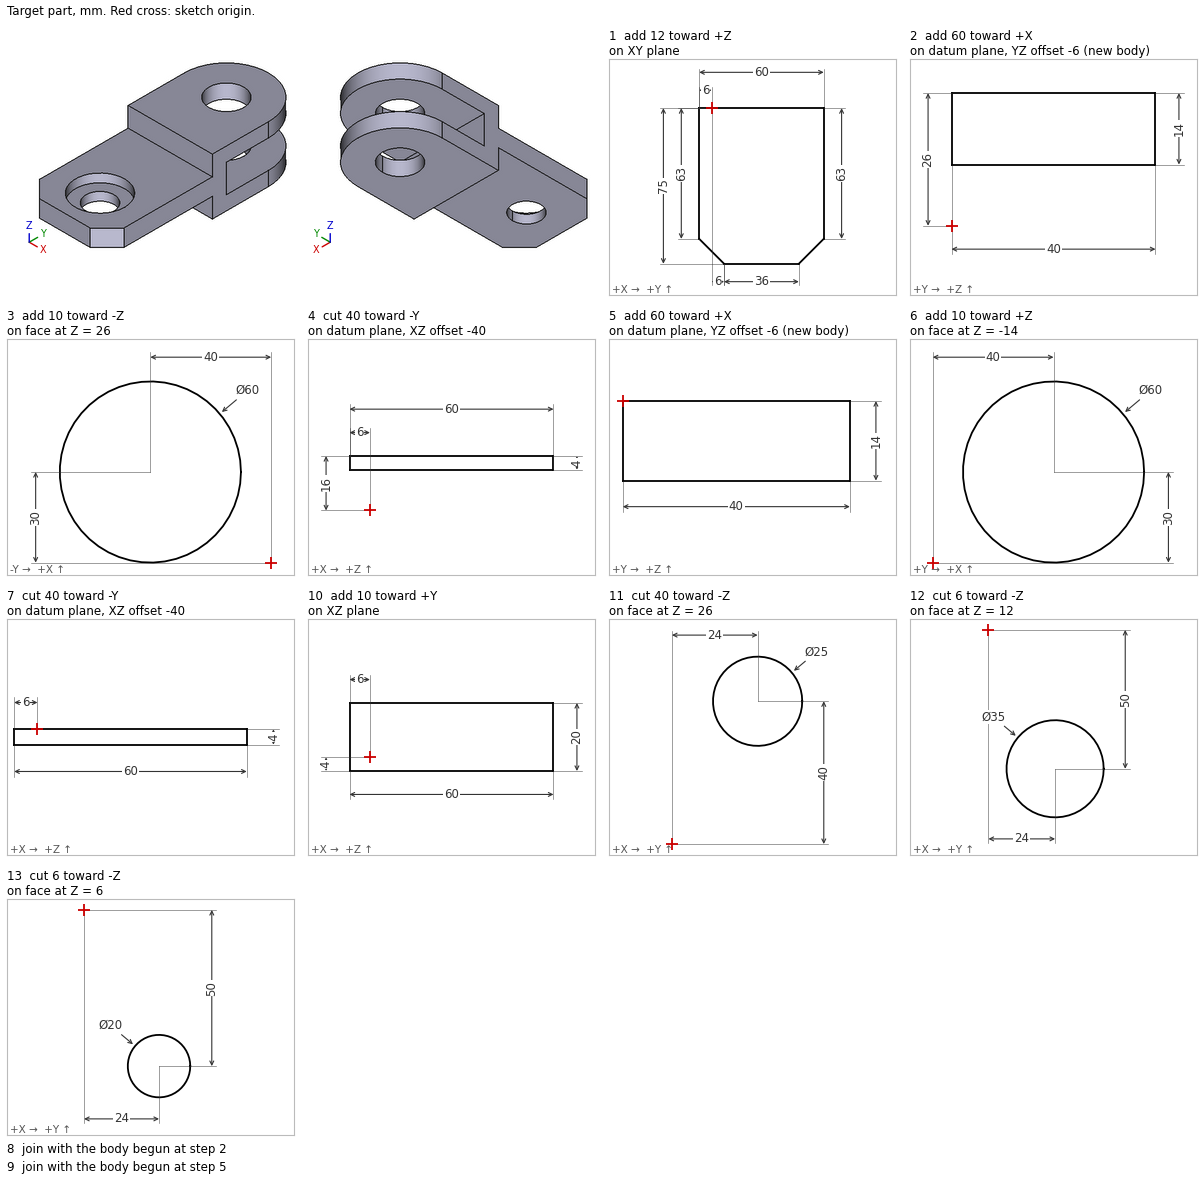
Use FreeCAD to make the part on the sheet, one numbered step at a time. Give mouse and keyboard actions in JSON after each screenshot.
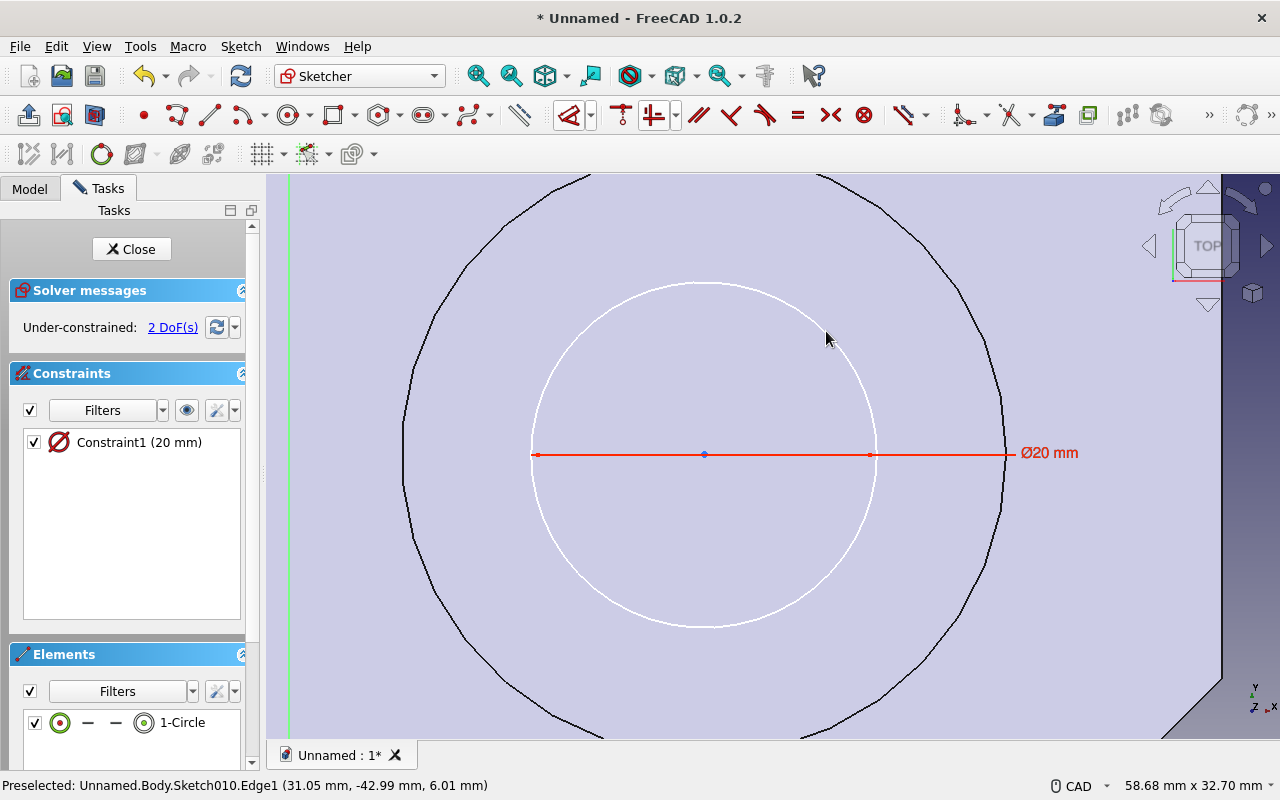
{"action": "left_click", "coordinate": [704, 455]}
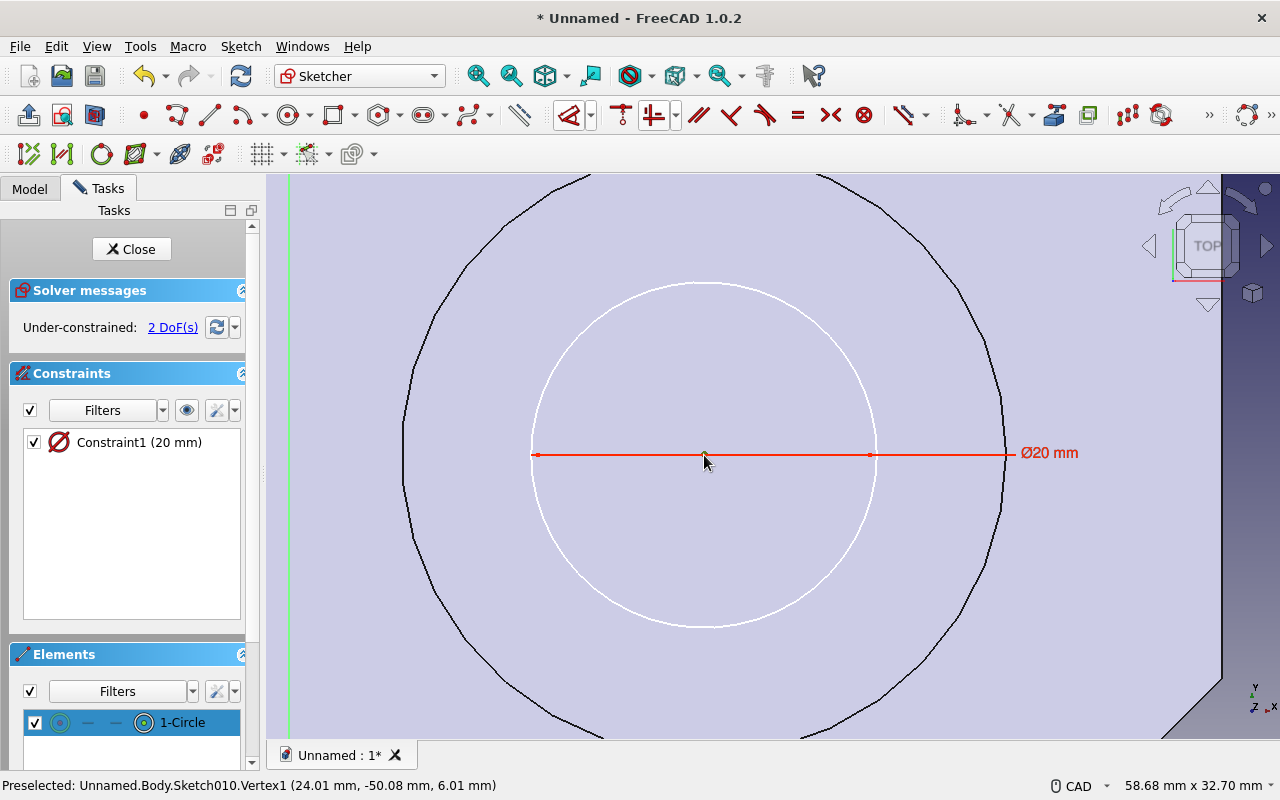
{"action": "left_click", "coordinate": [590, 116]}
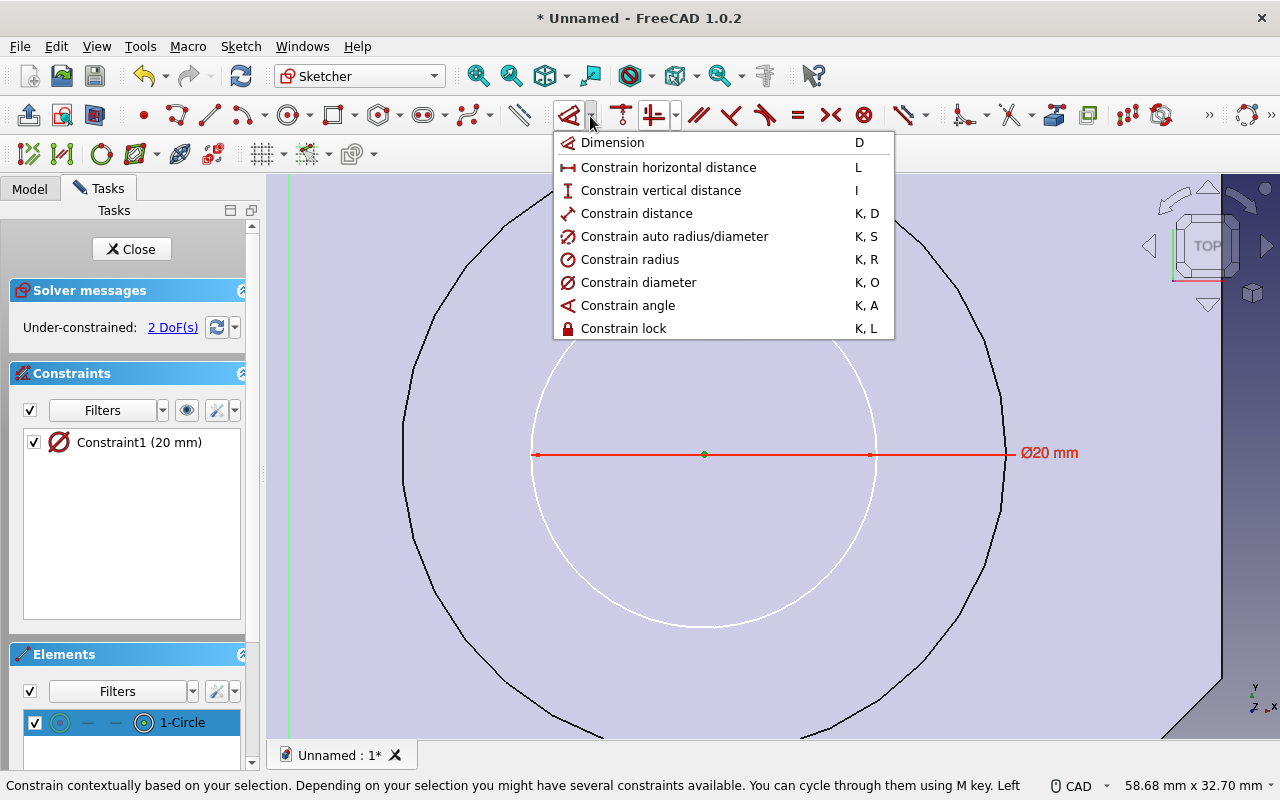
{"action": "left_click", "coordinate": [724, 168]}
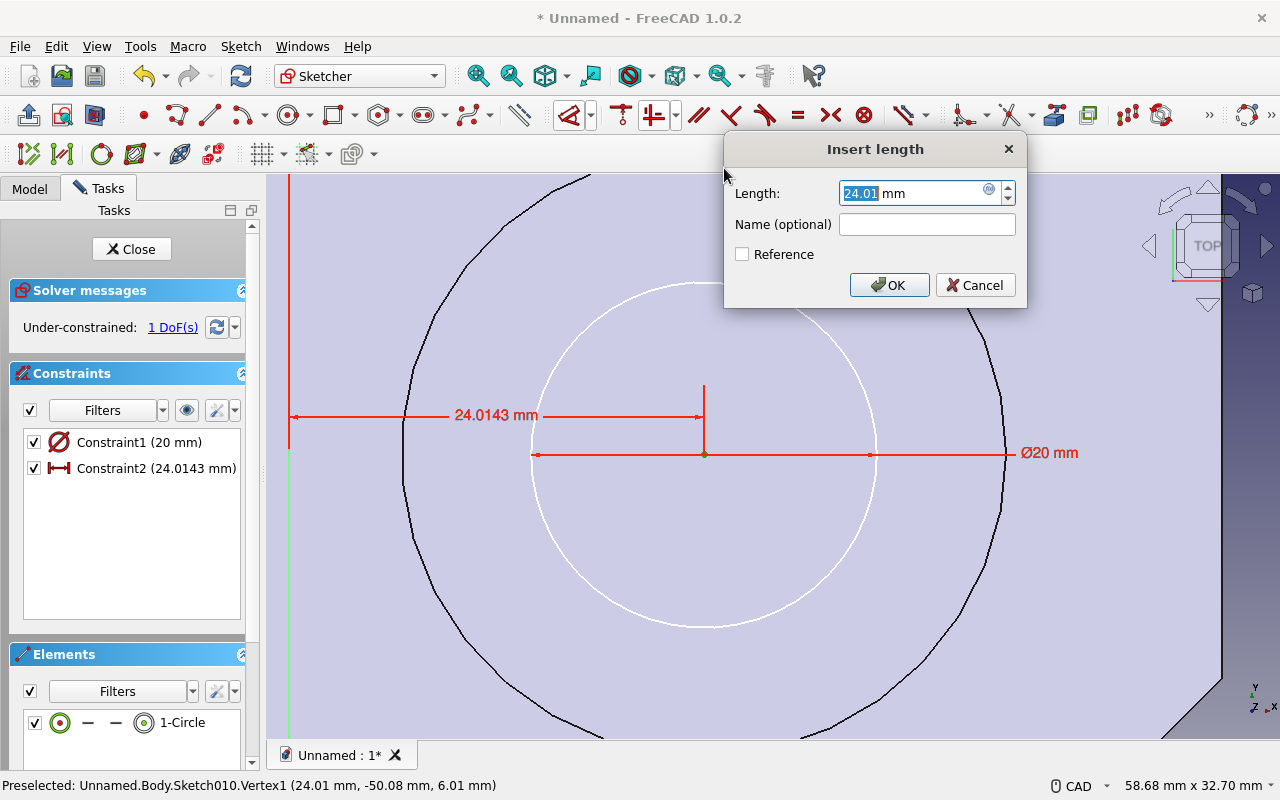
{"action": "type", "text": "24"}
{"action": "key", "text": "Return"}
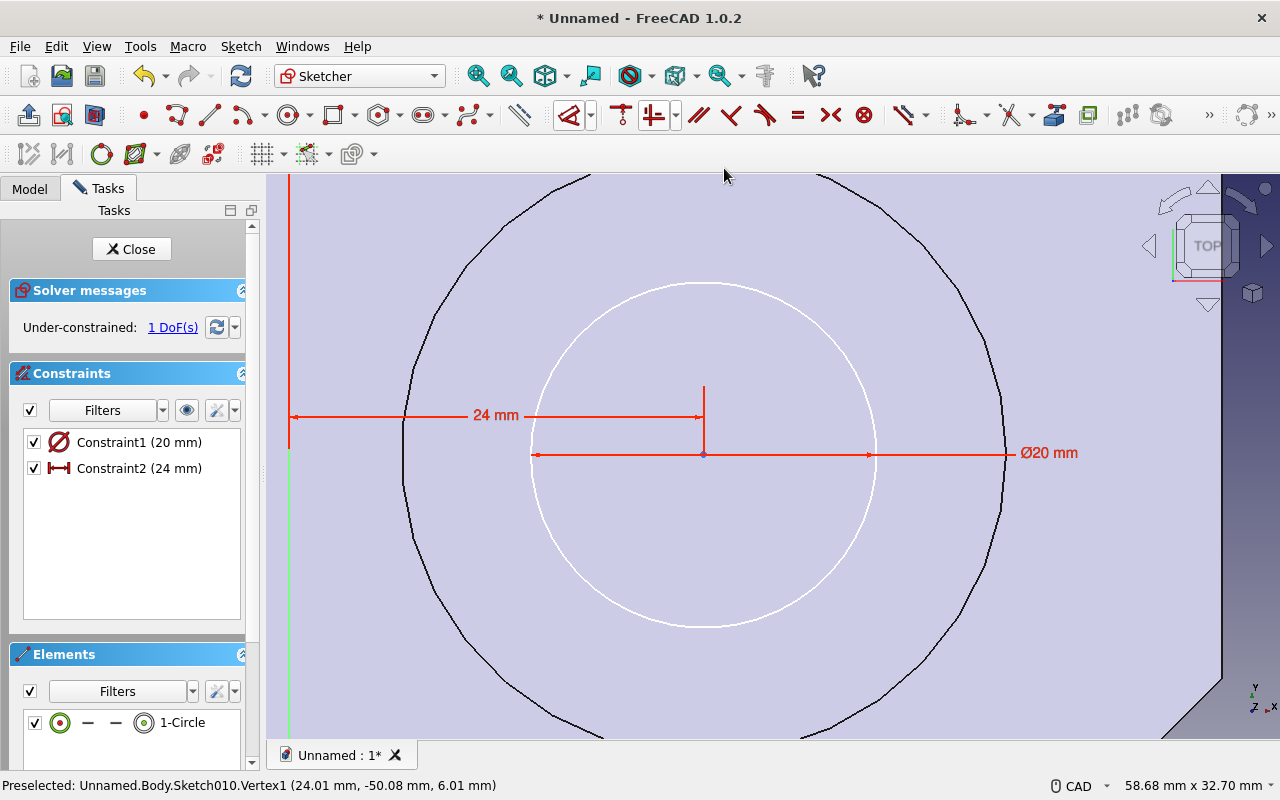
{"action": "left_click", "coordinate": [704, 455]}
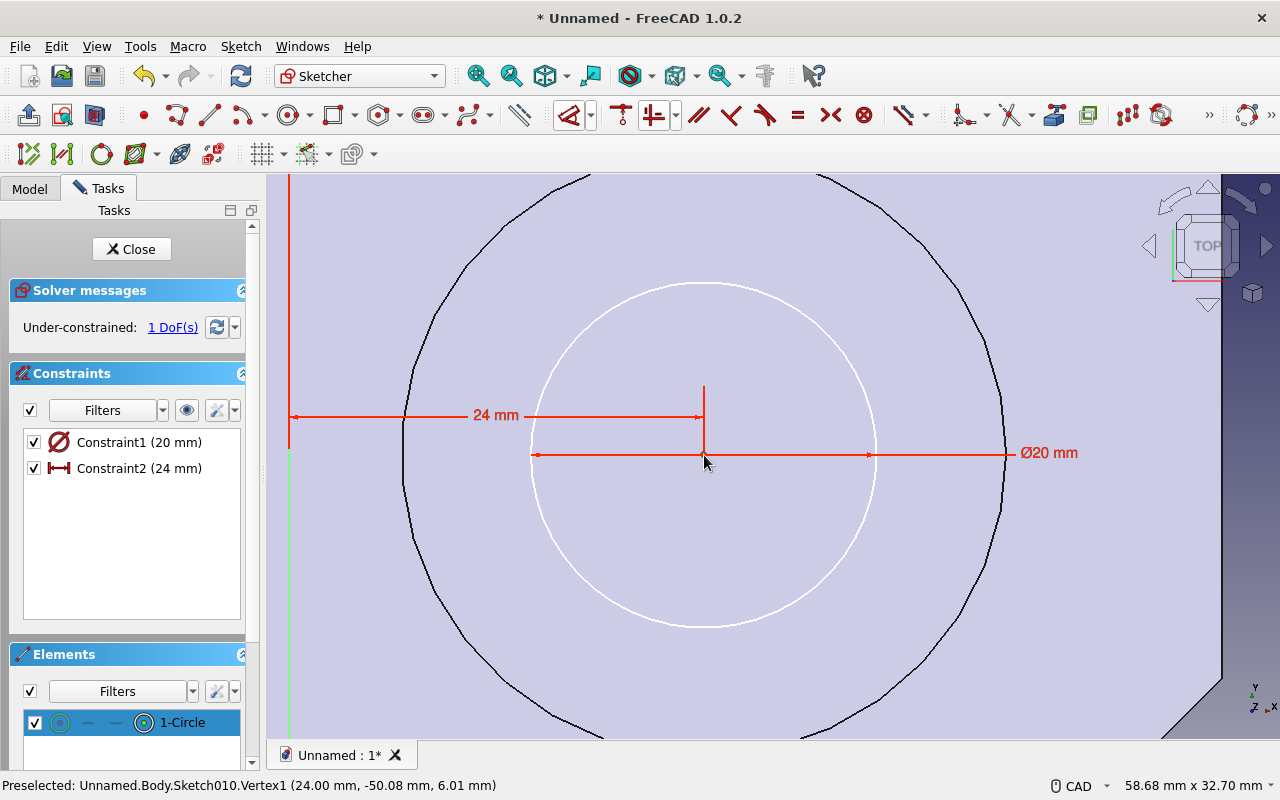
{"action": "left_click", "coordinate": [590, 116]}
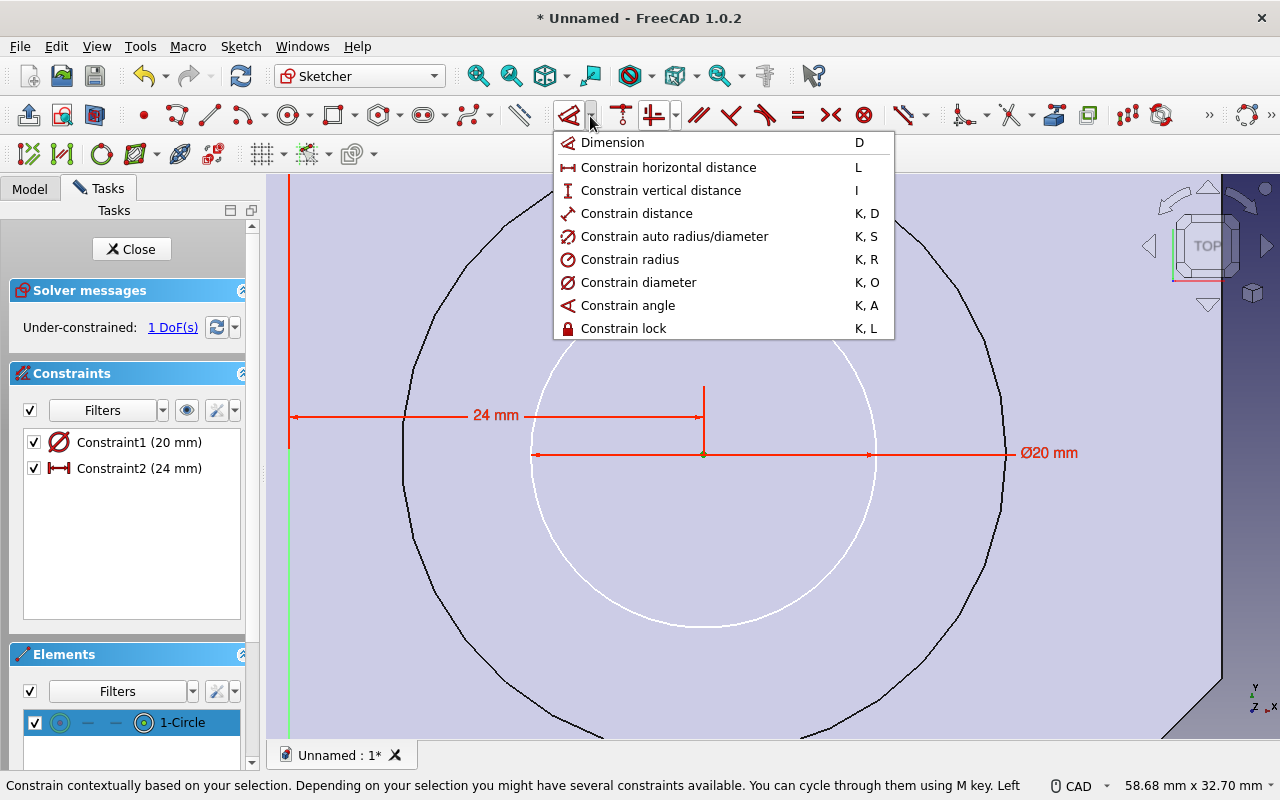
{"action": "left_click", "coordinate": [724, 190]}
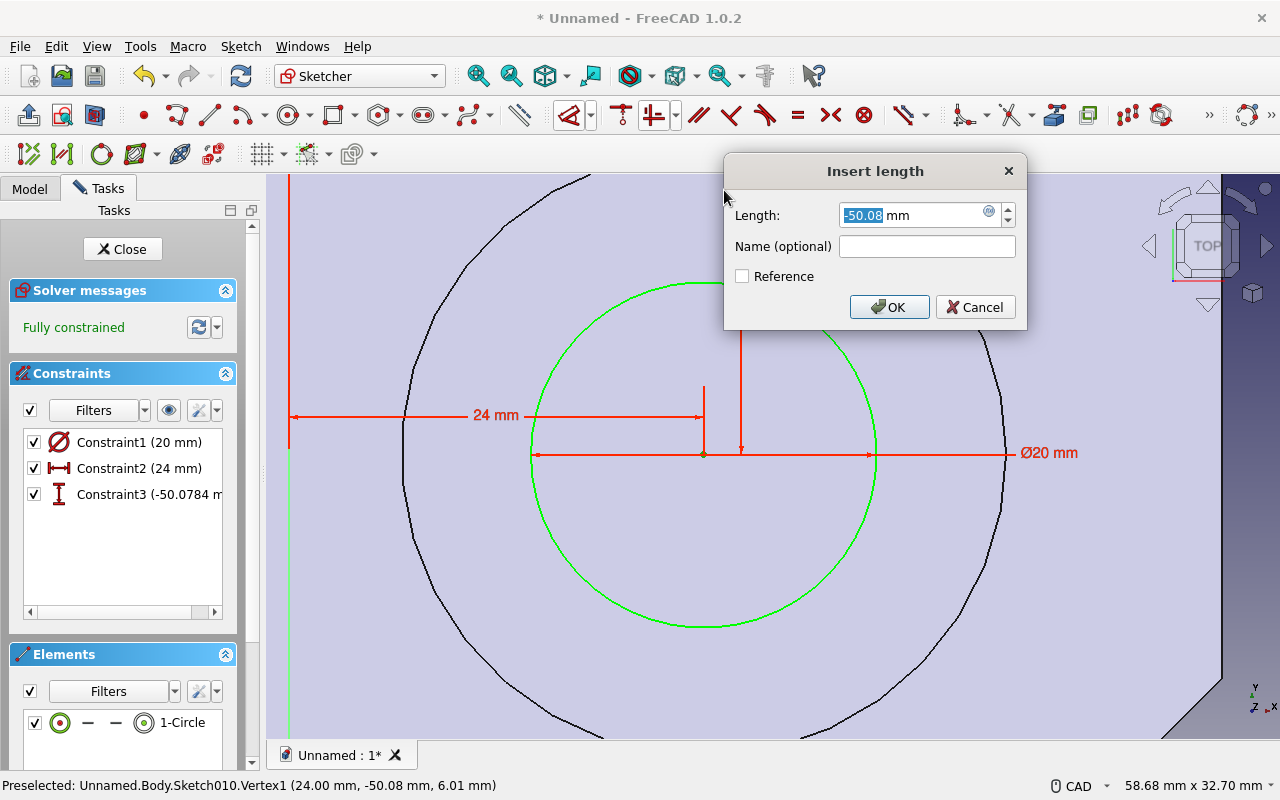
{"action": "type", "text": "-50"}
{"action": "key", "text": "Return"}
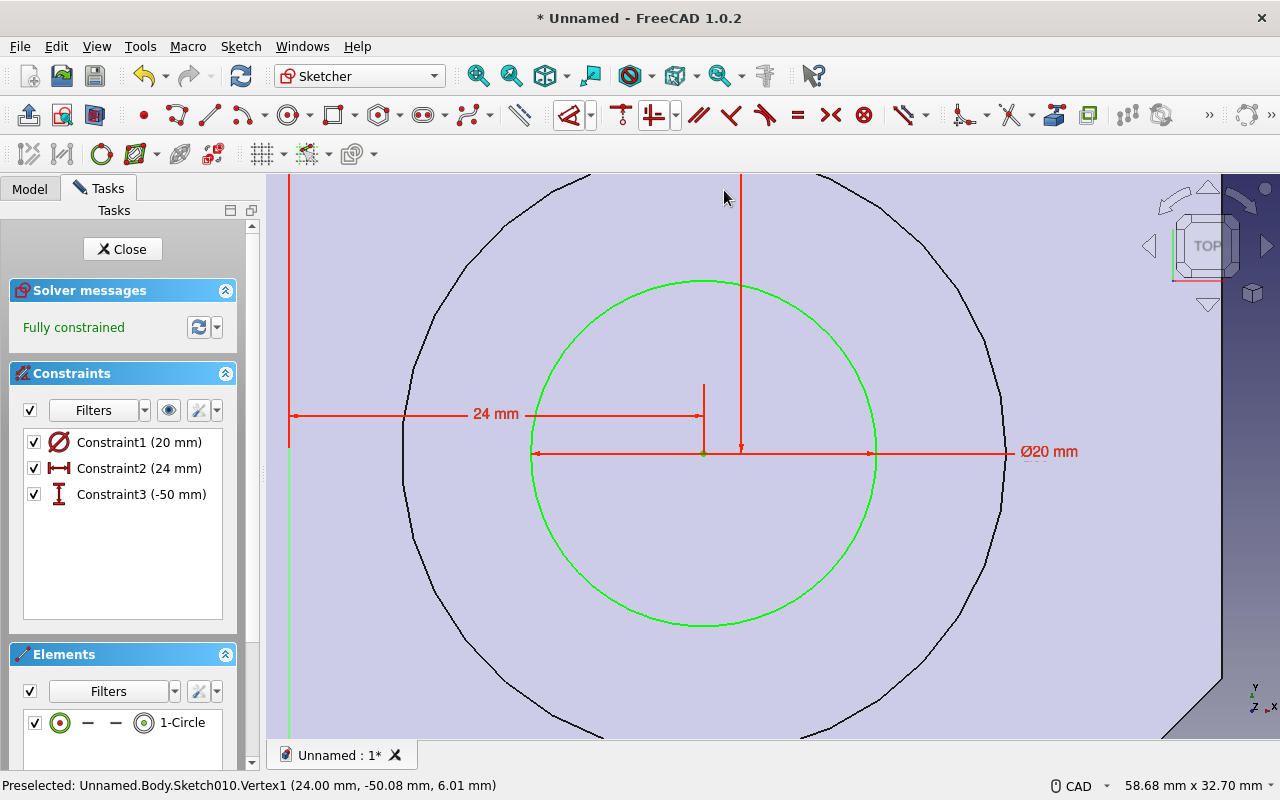
{"action": "left_click", "coordinate": [123, 249]}